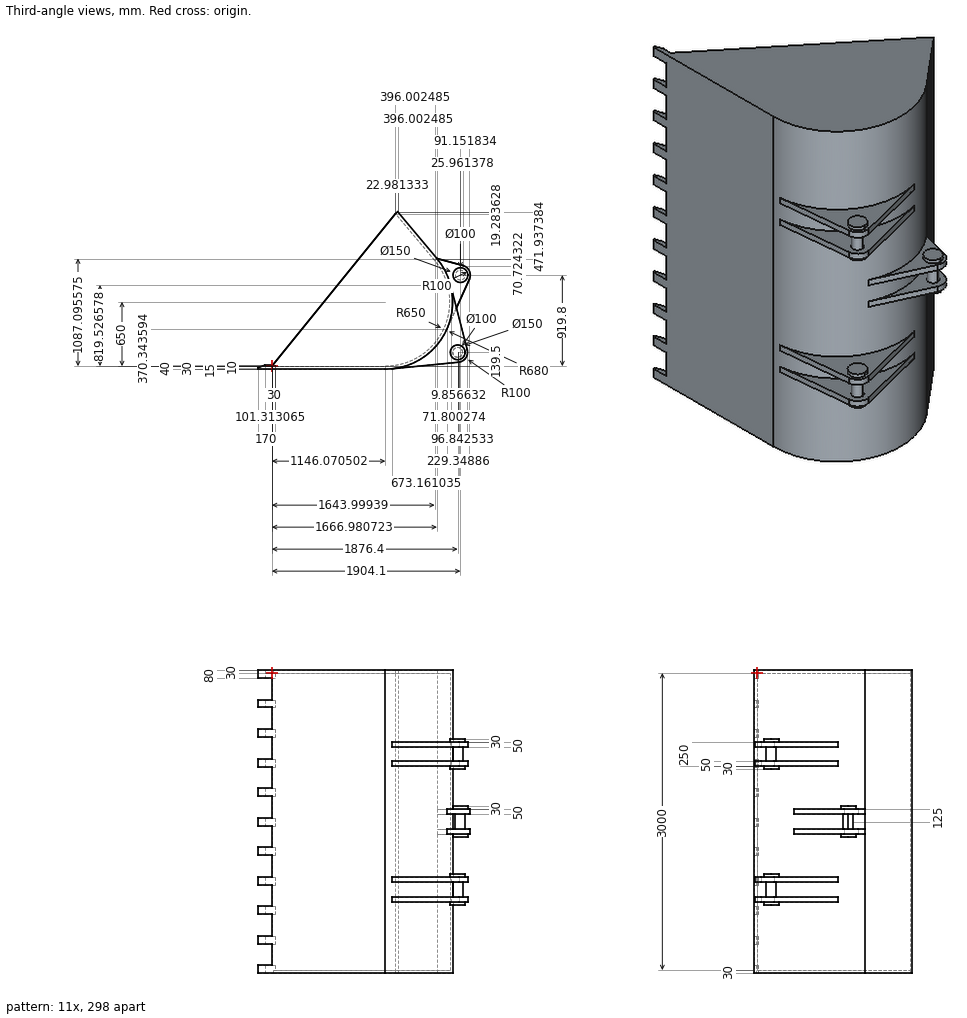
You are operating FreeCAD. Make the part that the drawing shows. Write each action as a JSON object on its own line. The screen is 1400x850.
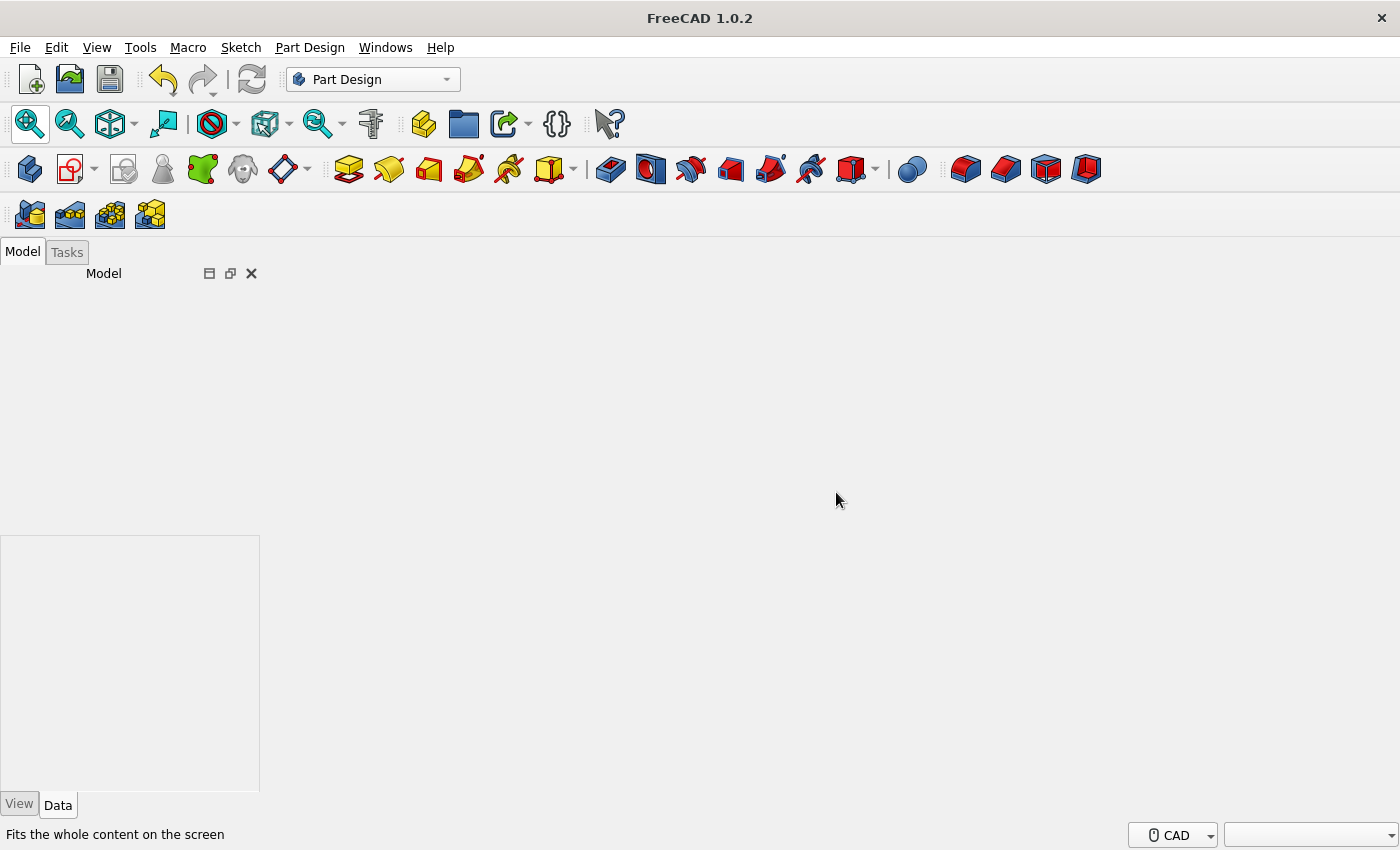
{"action": "left_click", "coordinate": [30, 80]}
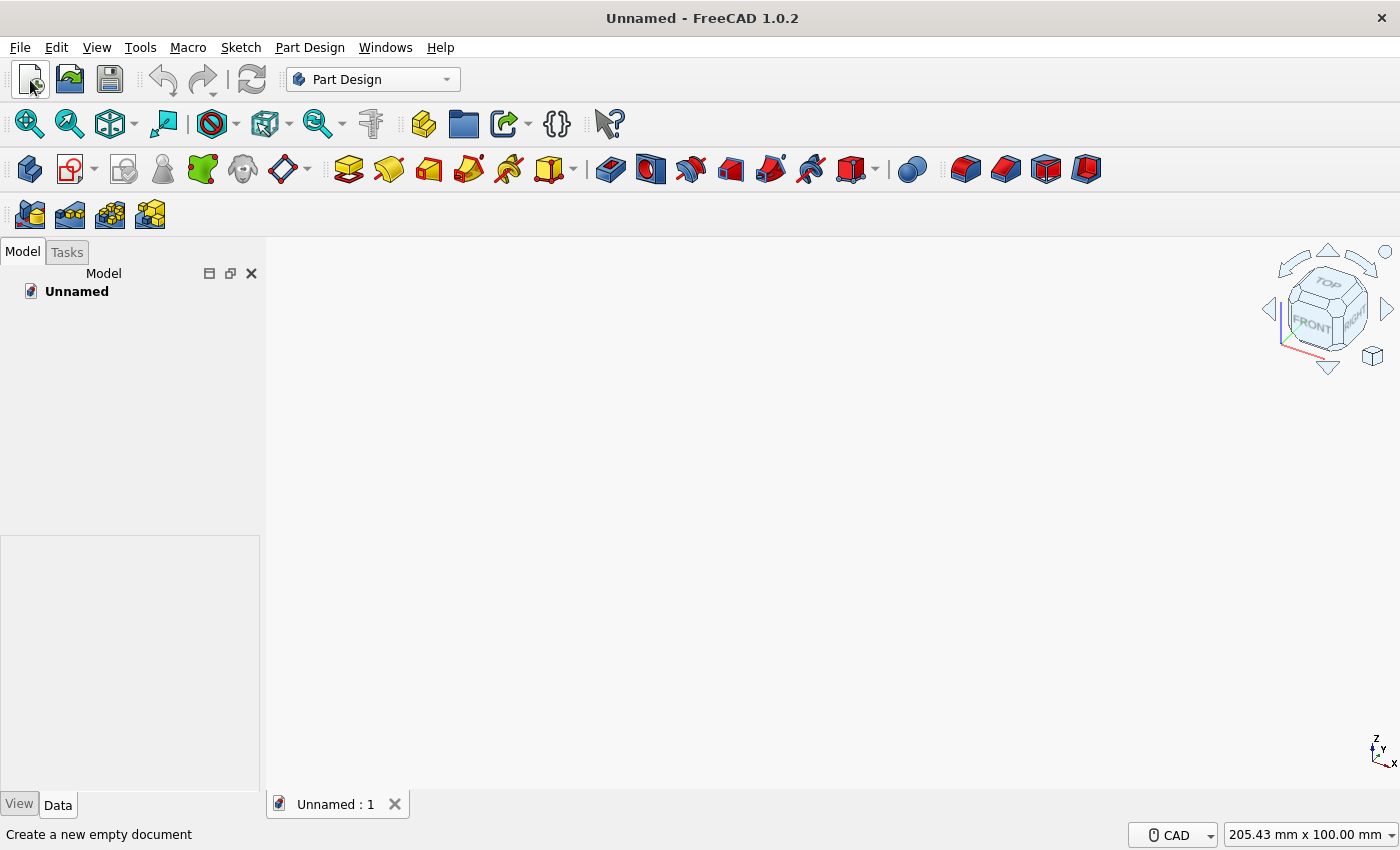
{"action": "left_click", "coordinate": [70, 170]}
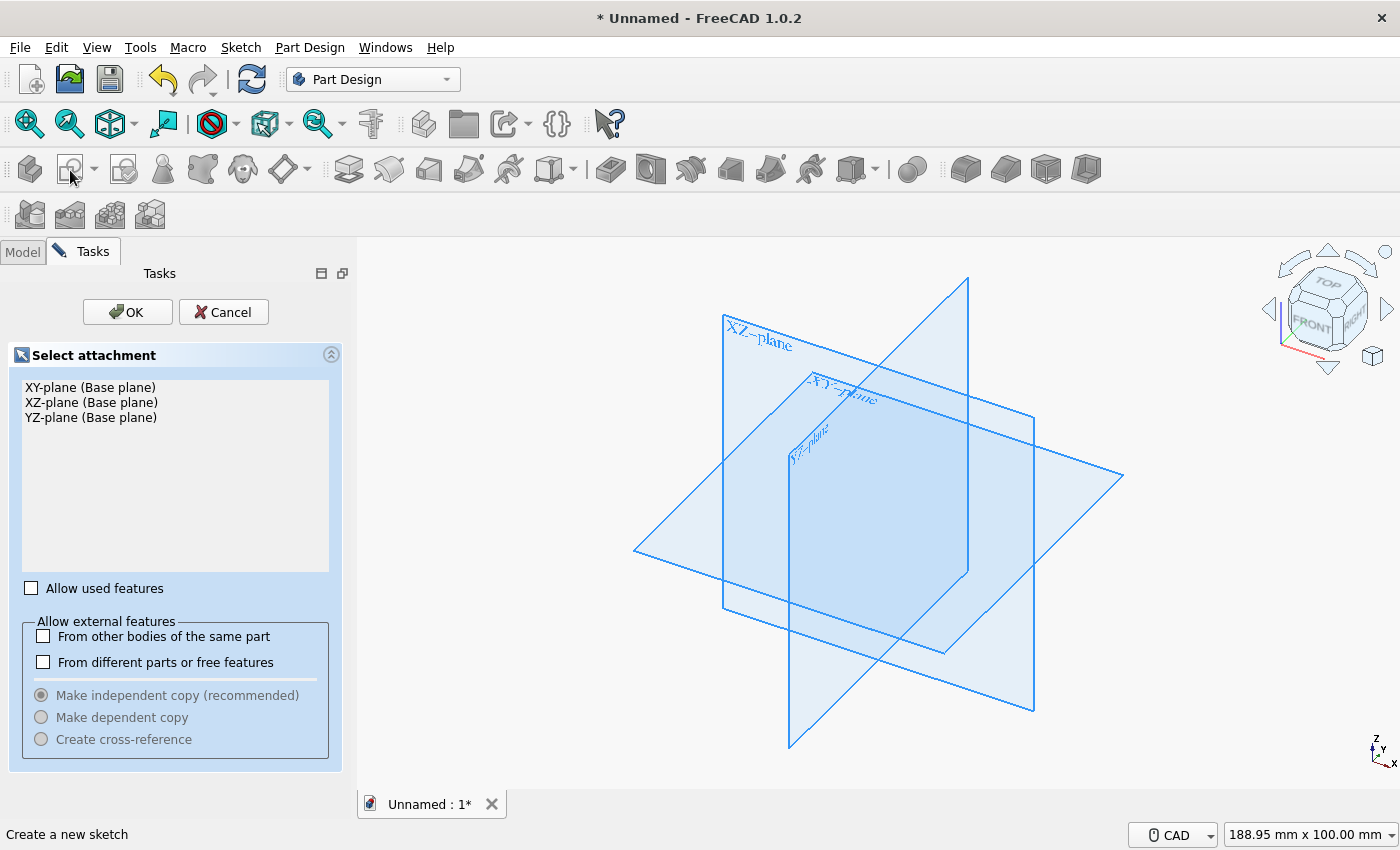
{"action": "left_click", "coordinate": [82, 388]}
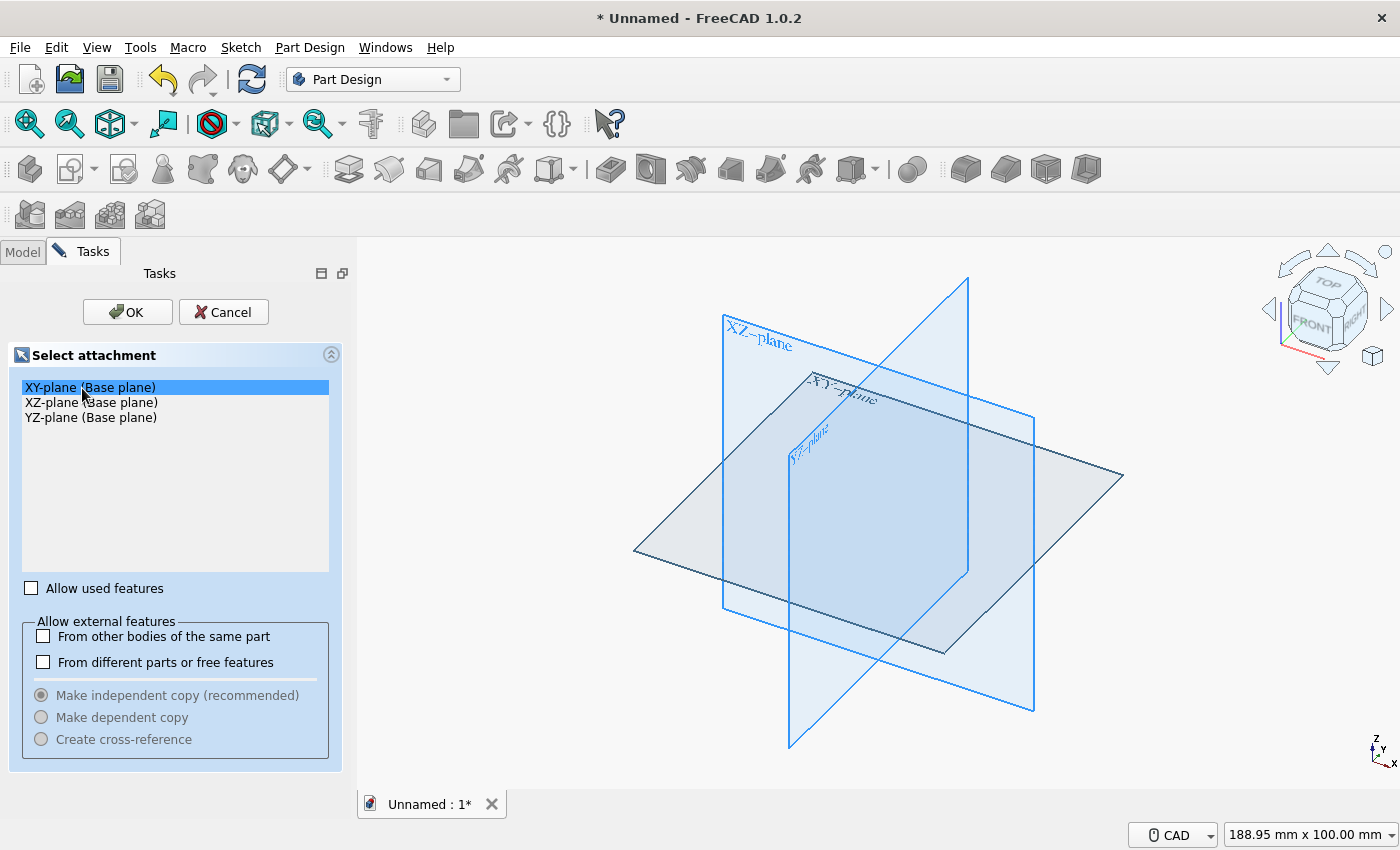
{"action": "left_click", "coordinate": [128, 312]}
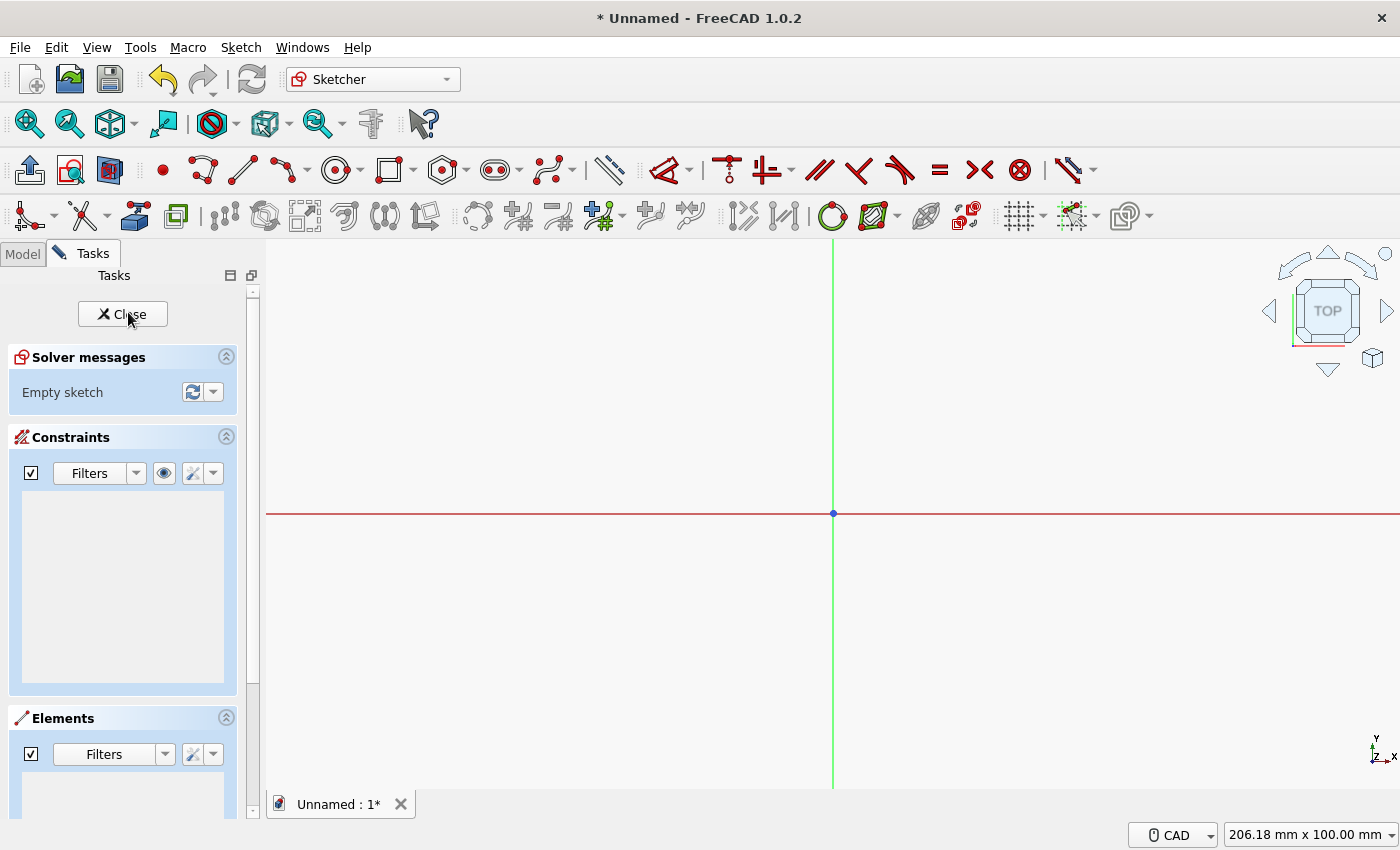
{"action": "scroll", "coordinate": [507, 734], "scroll_direction": "down", "scroll_amount": 15}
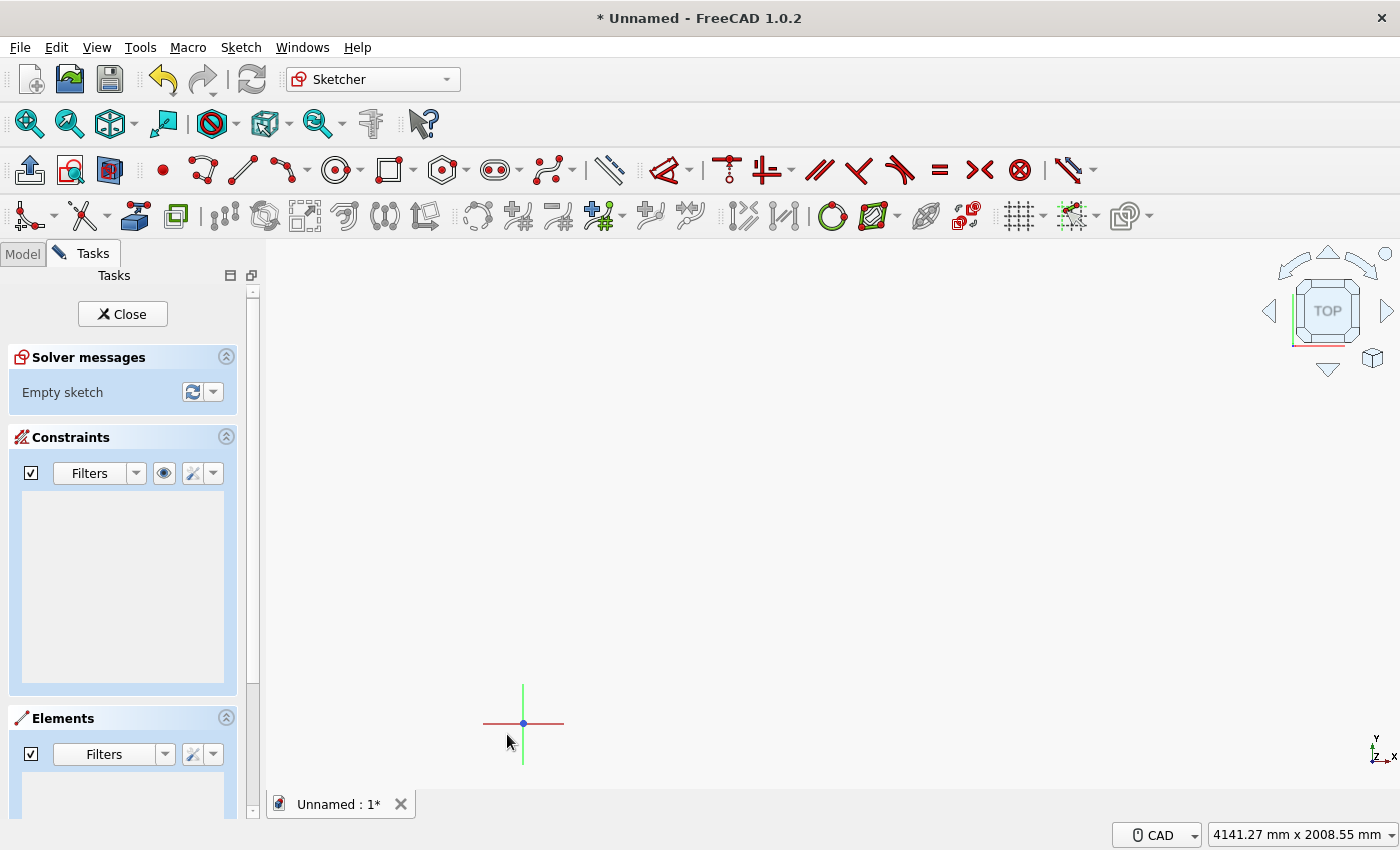
{"action": "left_click", "coordinate": [204, 170]}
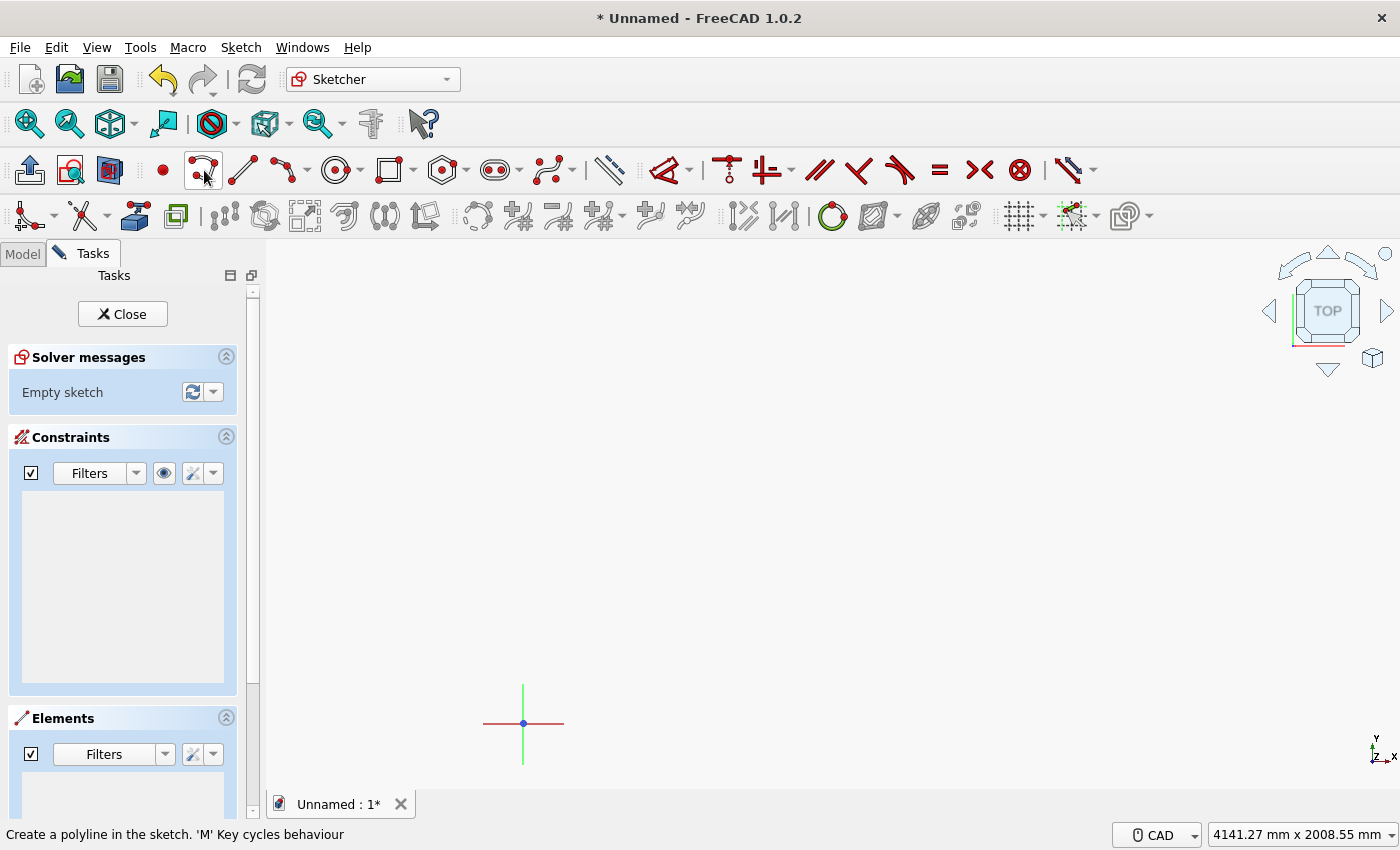
{"action": "left_click", "coordinate": [980, 426]}
{"action": "left_click", "coordinate": [871, 297]}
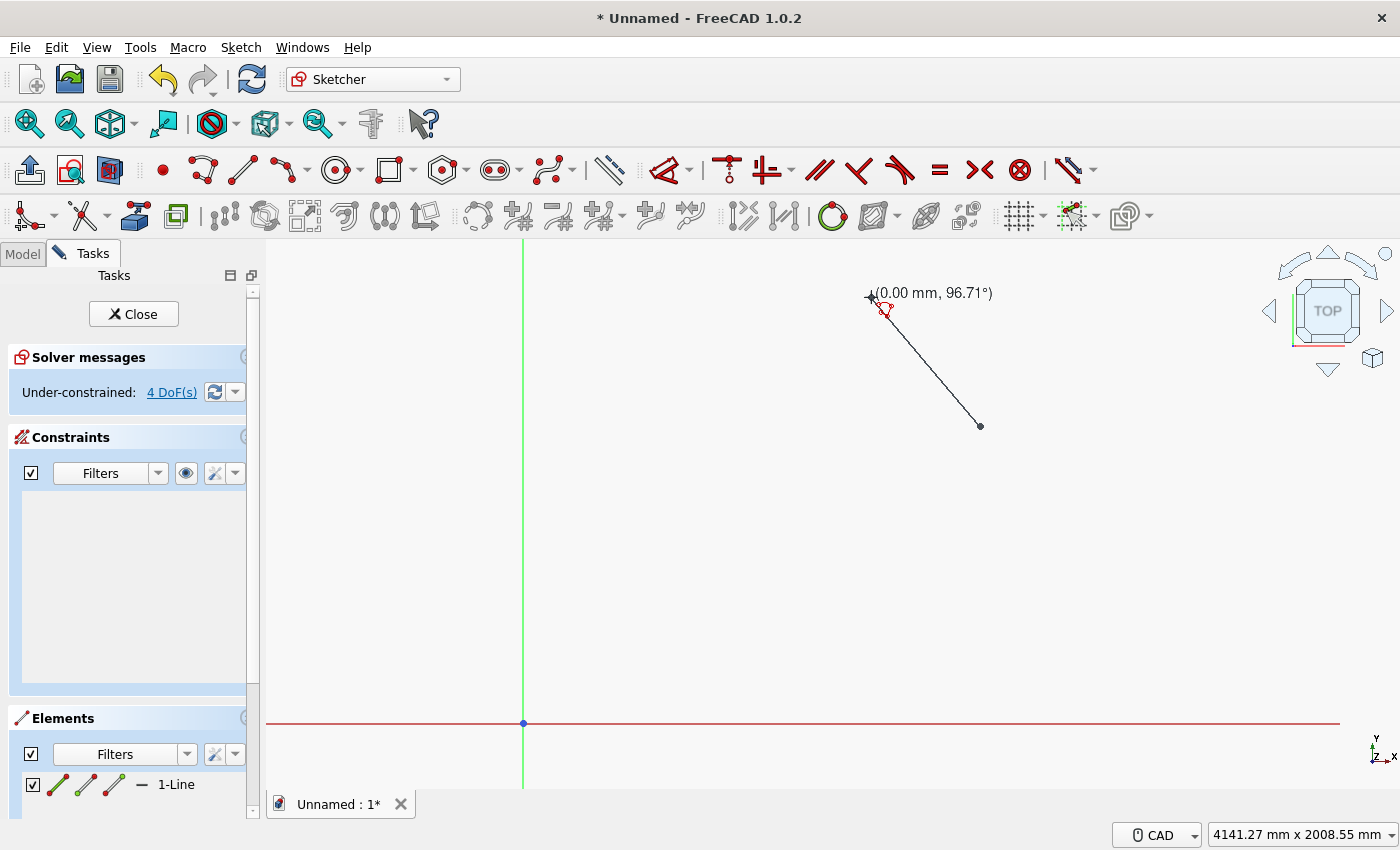
{"action": "scroll", "coordinate": [865, 302], "scroll_direction": "up", "scroll_amount": 4}